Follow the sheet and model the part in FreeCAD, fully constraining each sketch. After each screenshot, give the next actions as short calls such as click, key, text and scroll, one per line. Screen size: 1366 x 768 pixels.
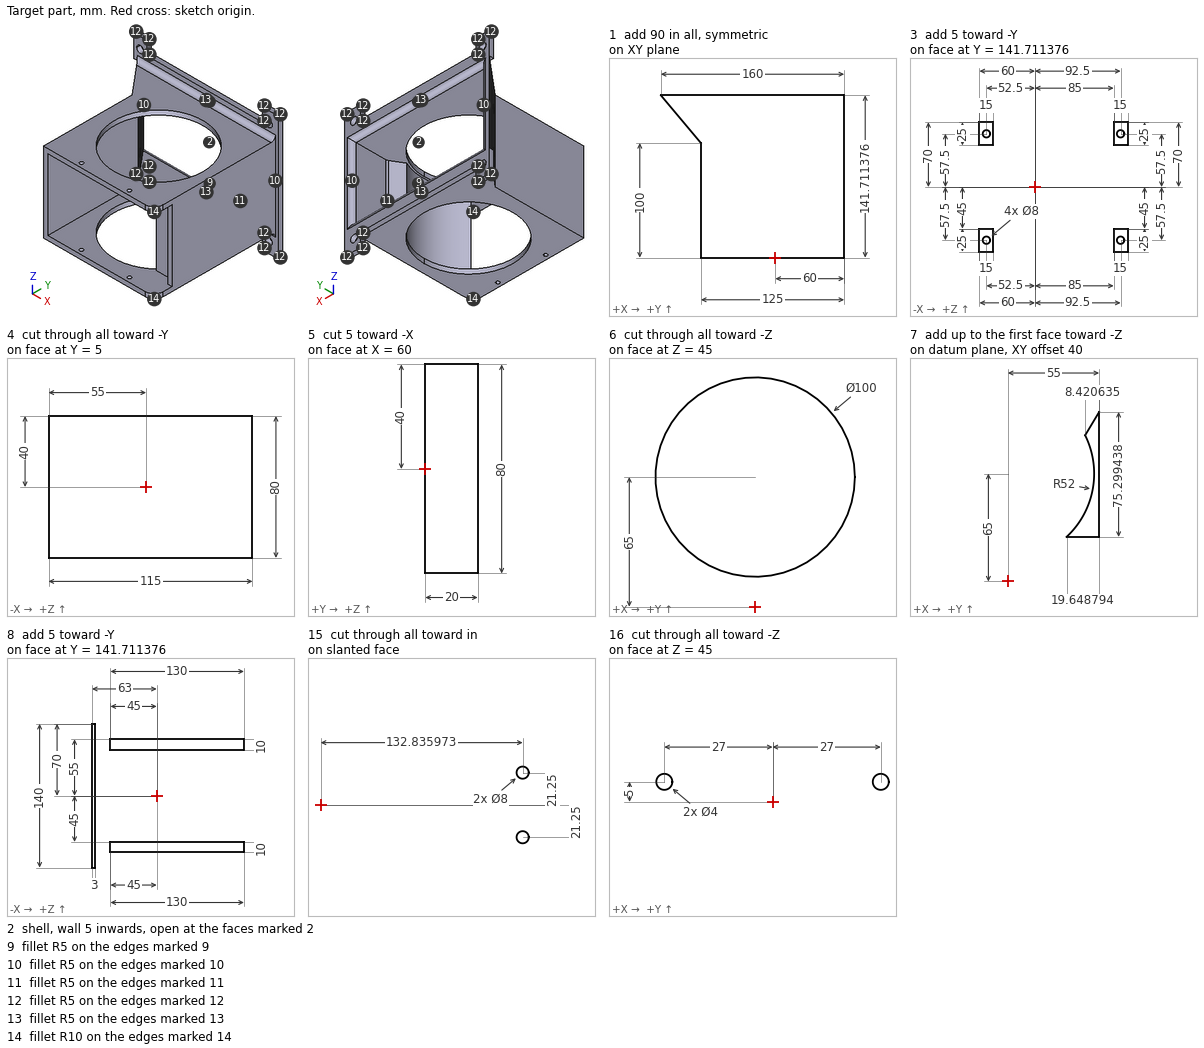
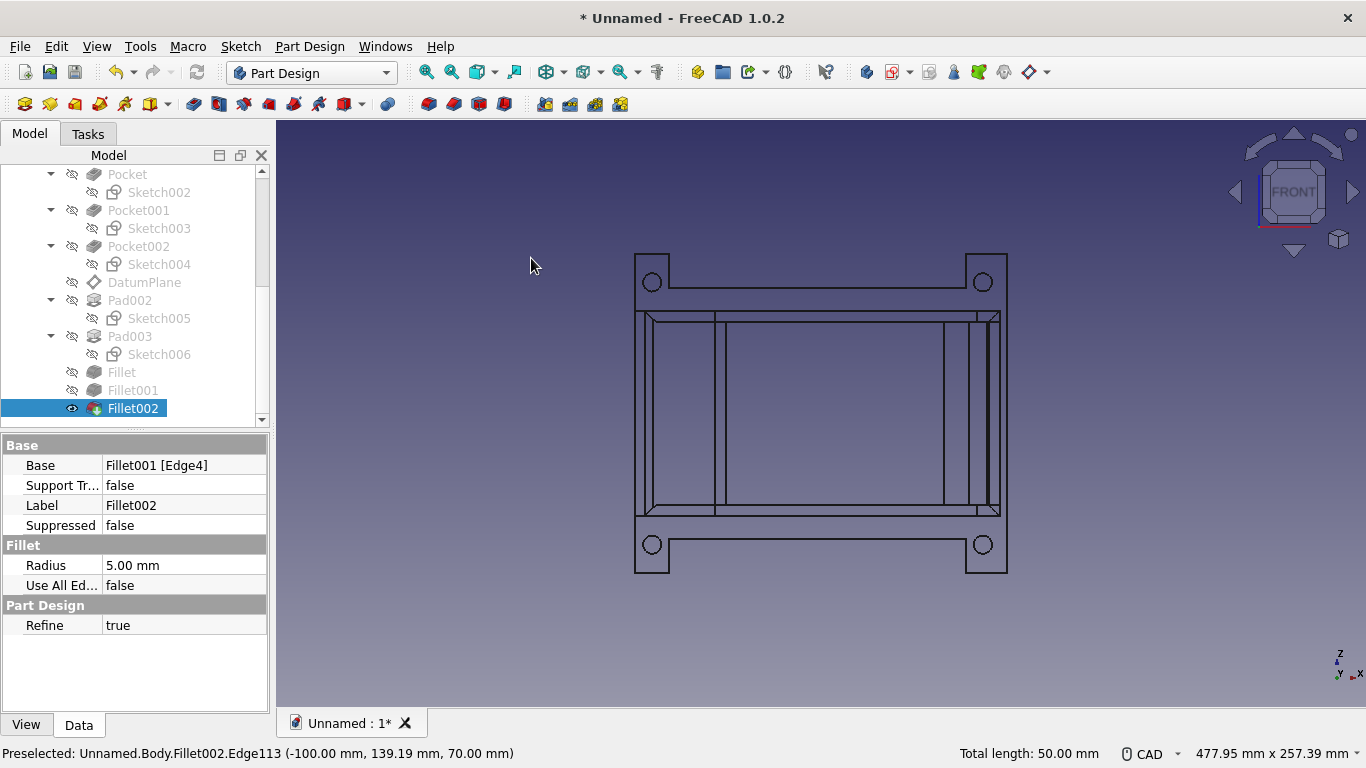
scroll(669, 572, up, 7)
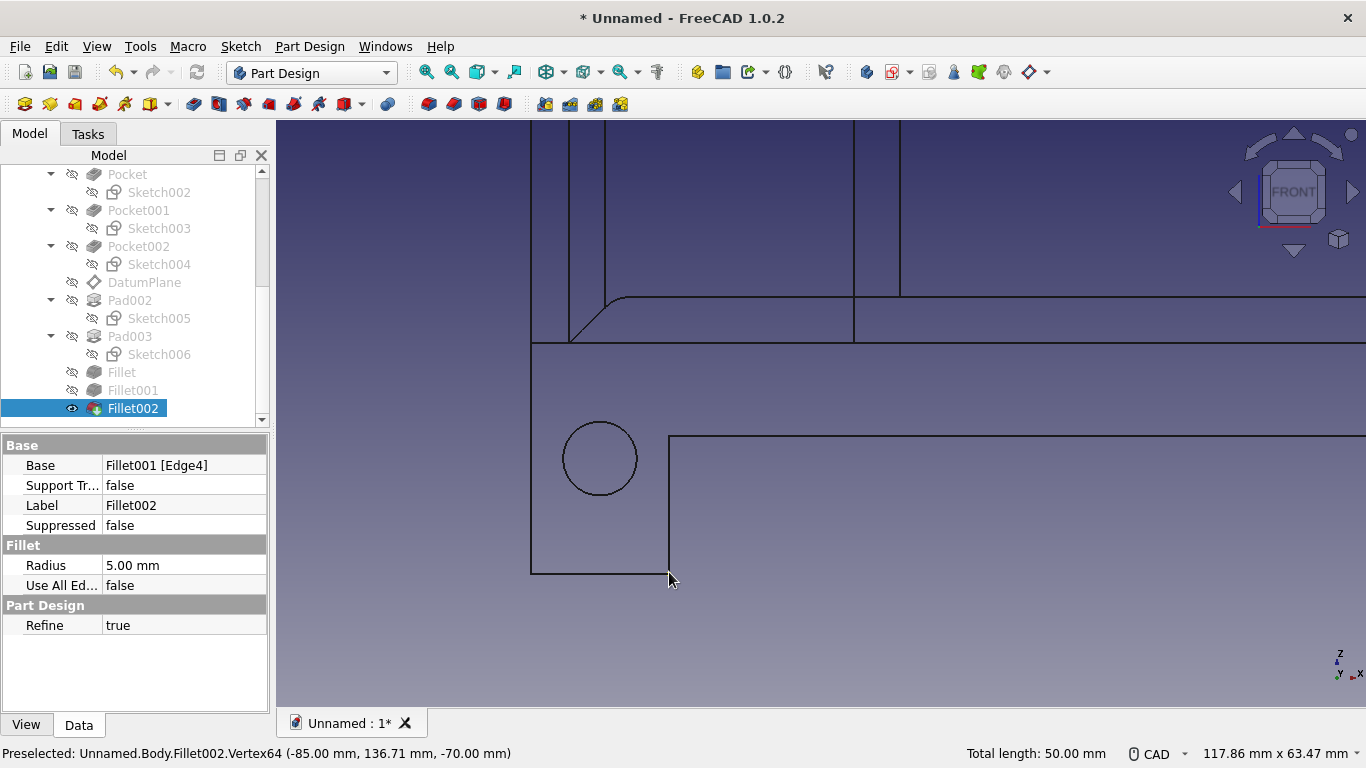
key(v)
key(f)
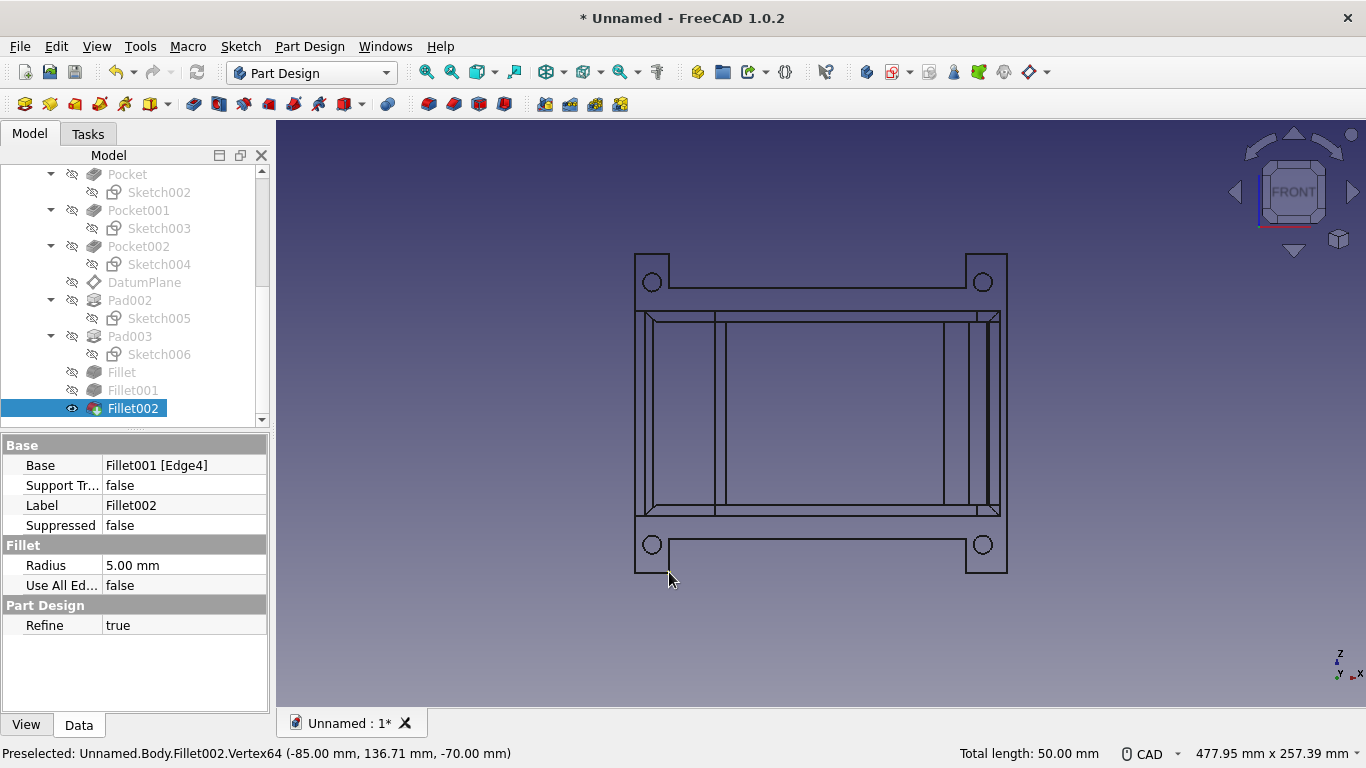
key(3)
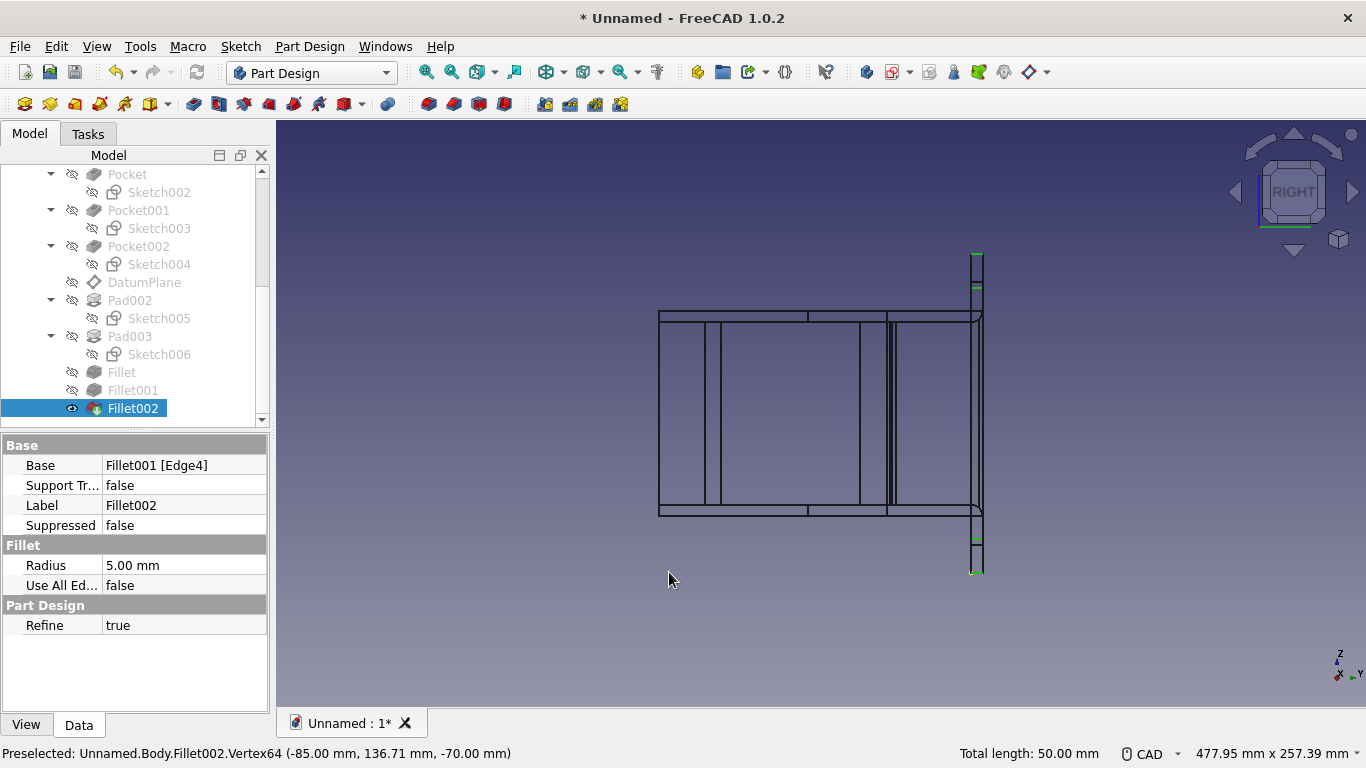
scroll(977, 572, up, 7)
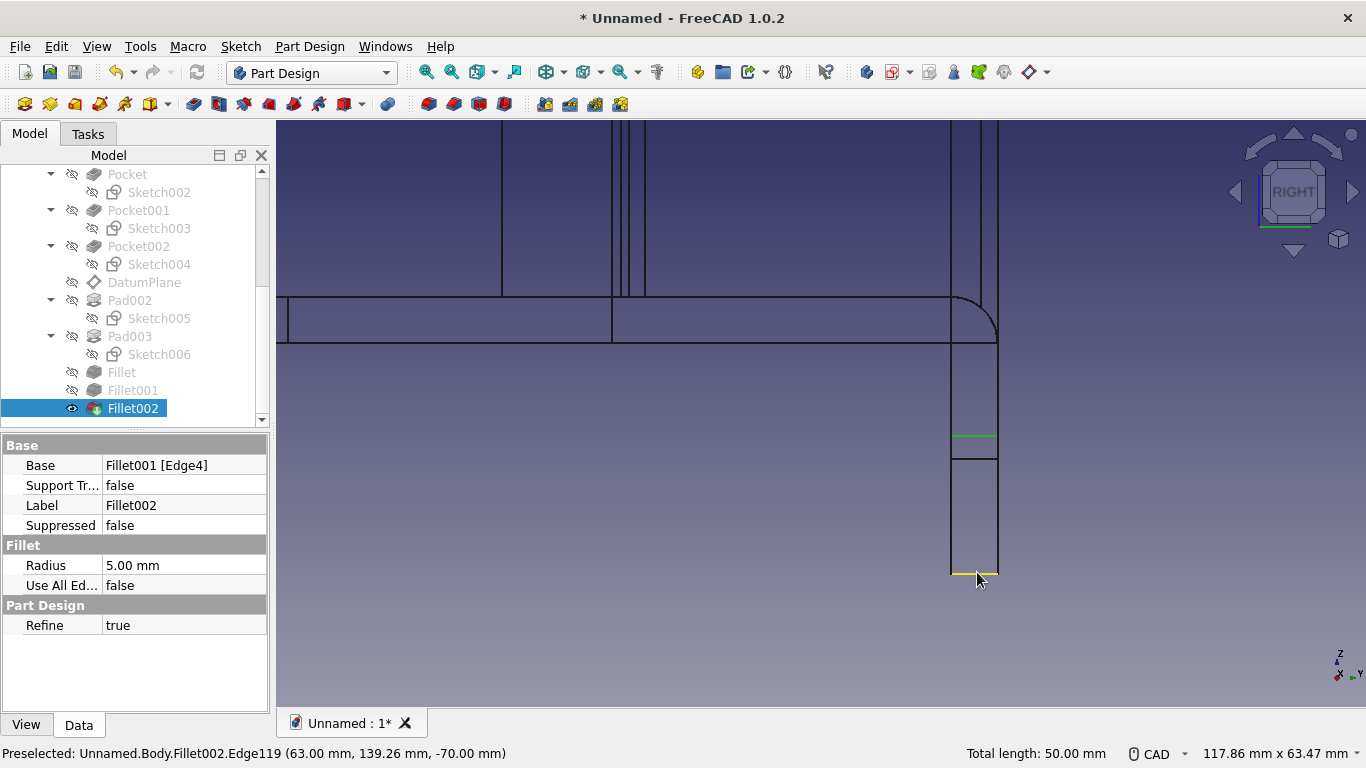
key(v)
key(f)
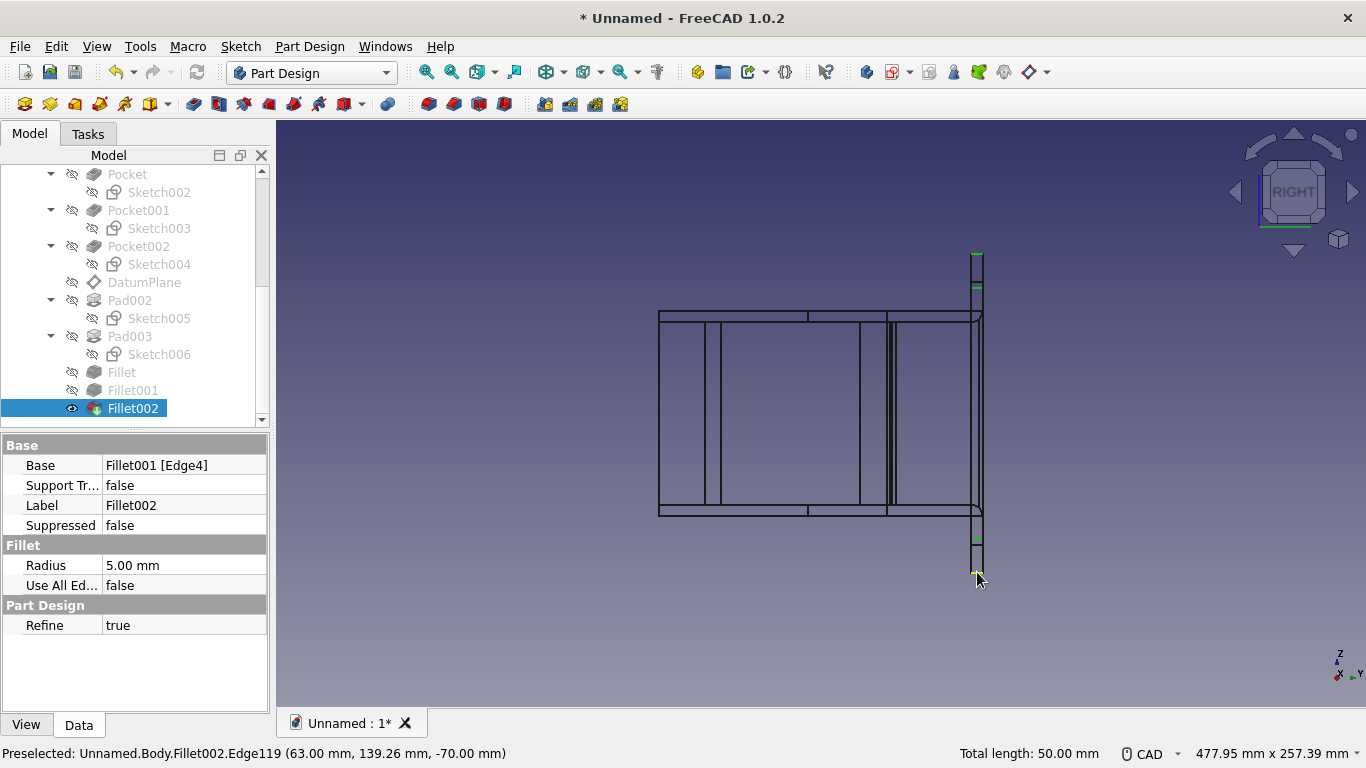
key(5)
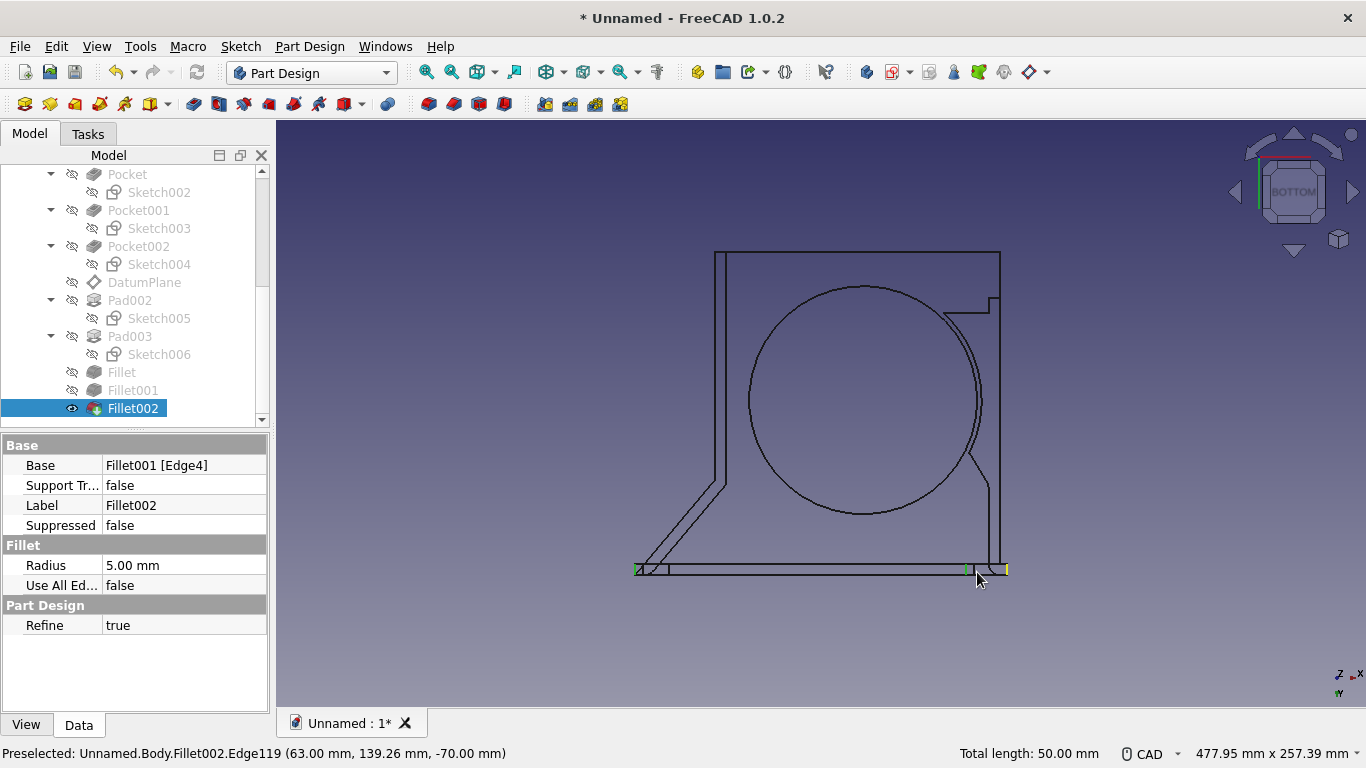
scroll(669, 568, up, 7)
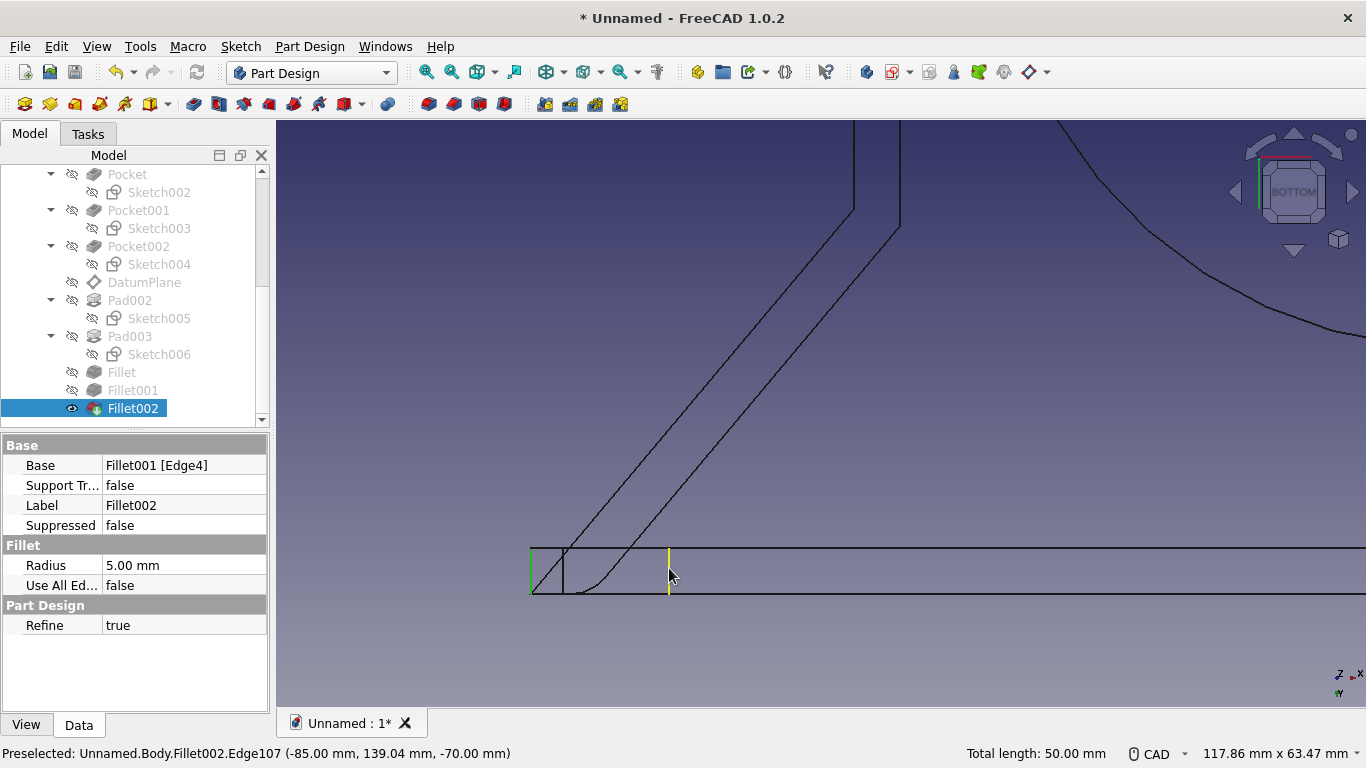
click(669, 570, ctrl)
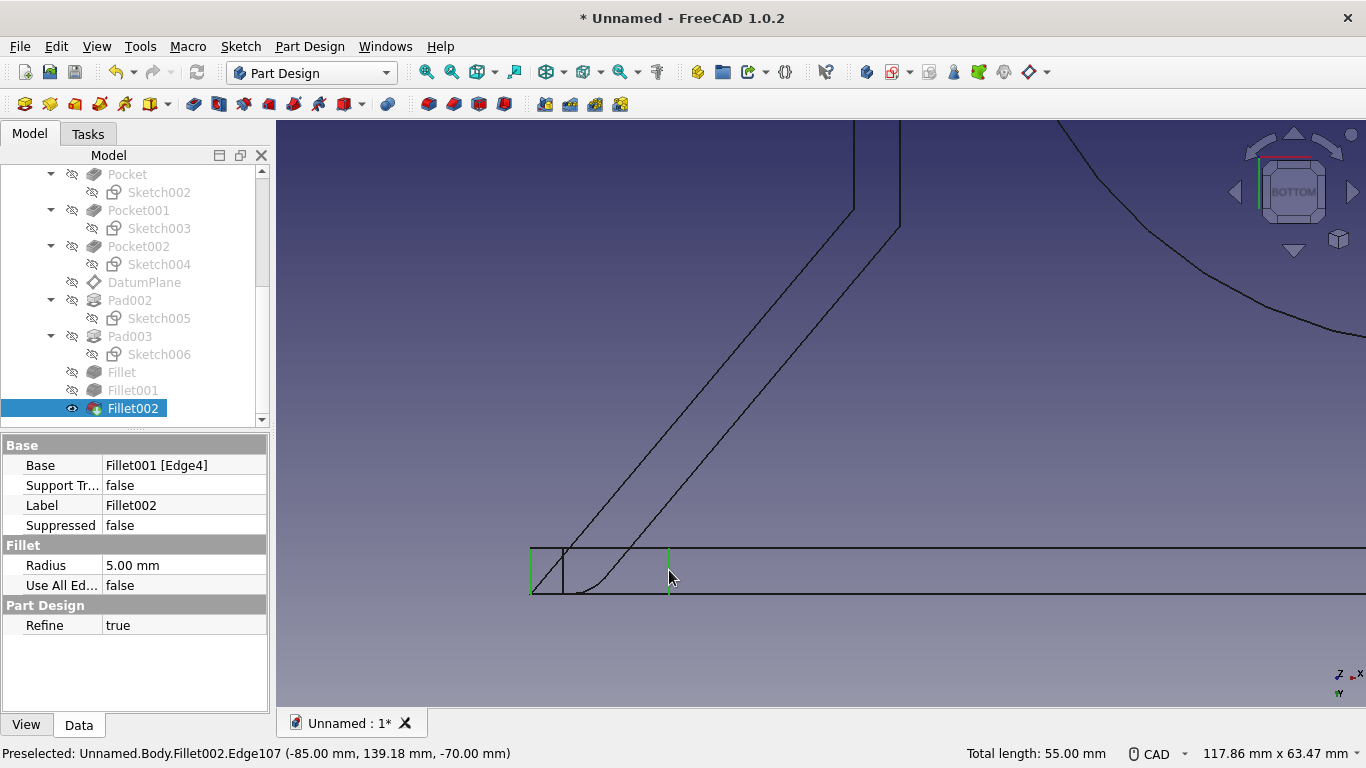
key(v)
key(f)